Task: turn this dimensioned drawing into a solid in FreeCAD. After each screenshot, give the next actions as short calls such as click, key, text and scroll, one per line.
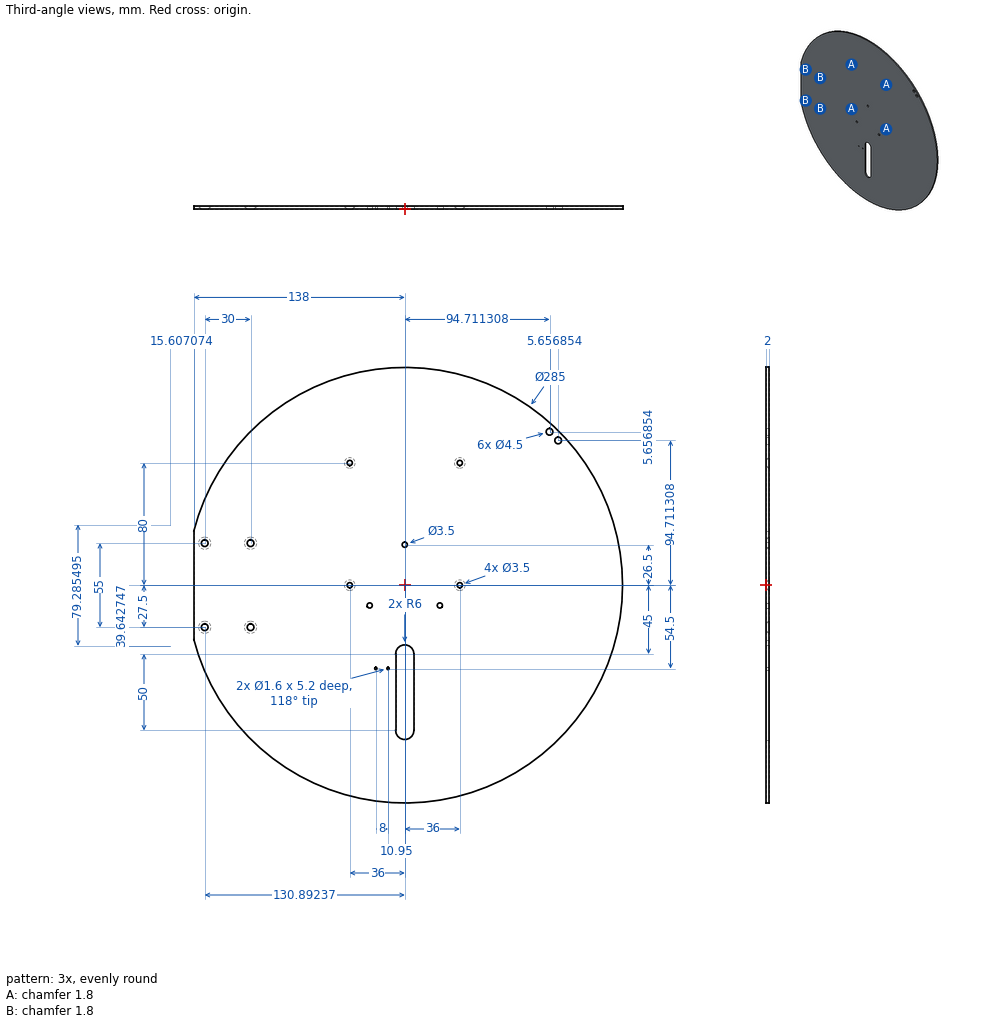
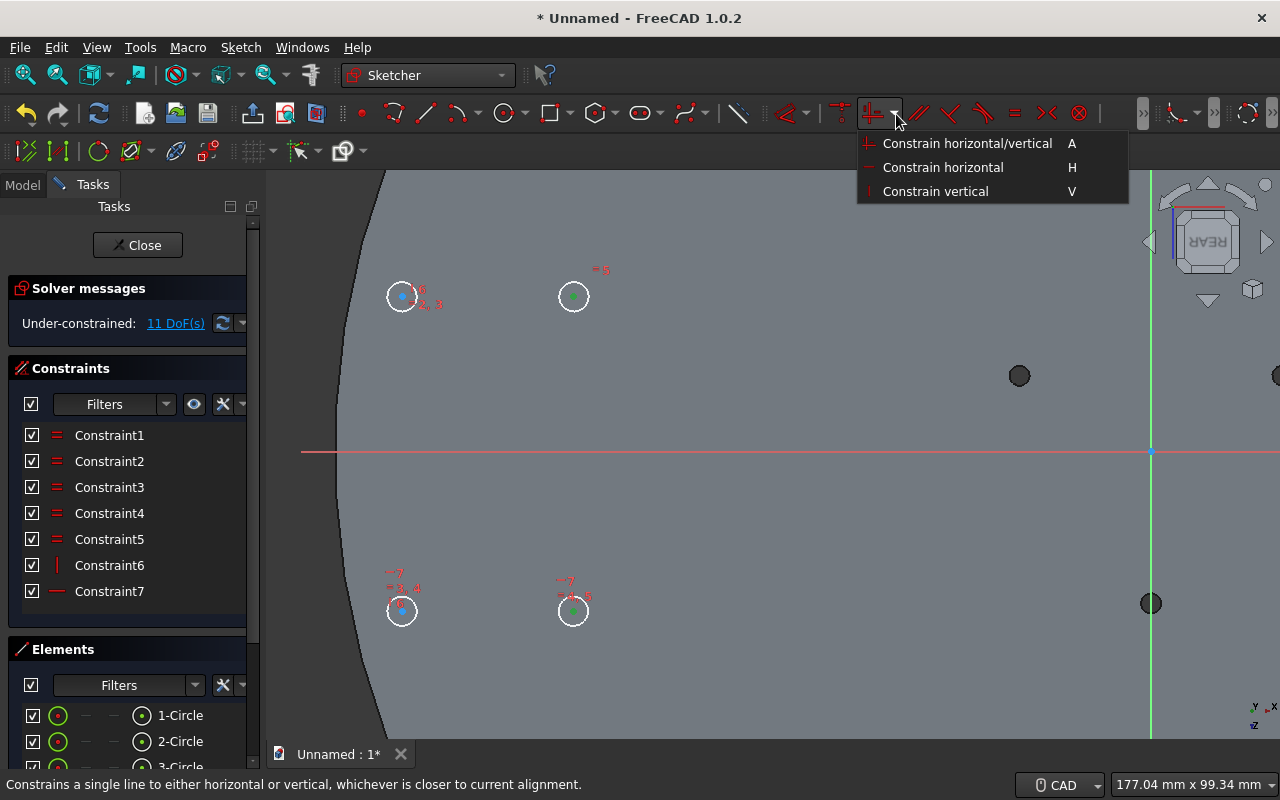
click(993, 191)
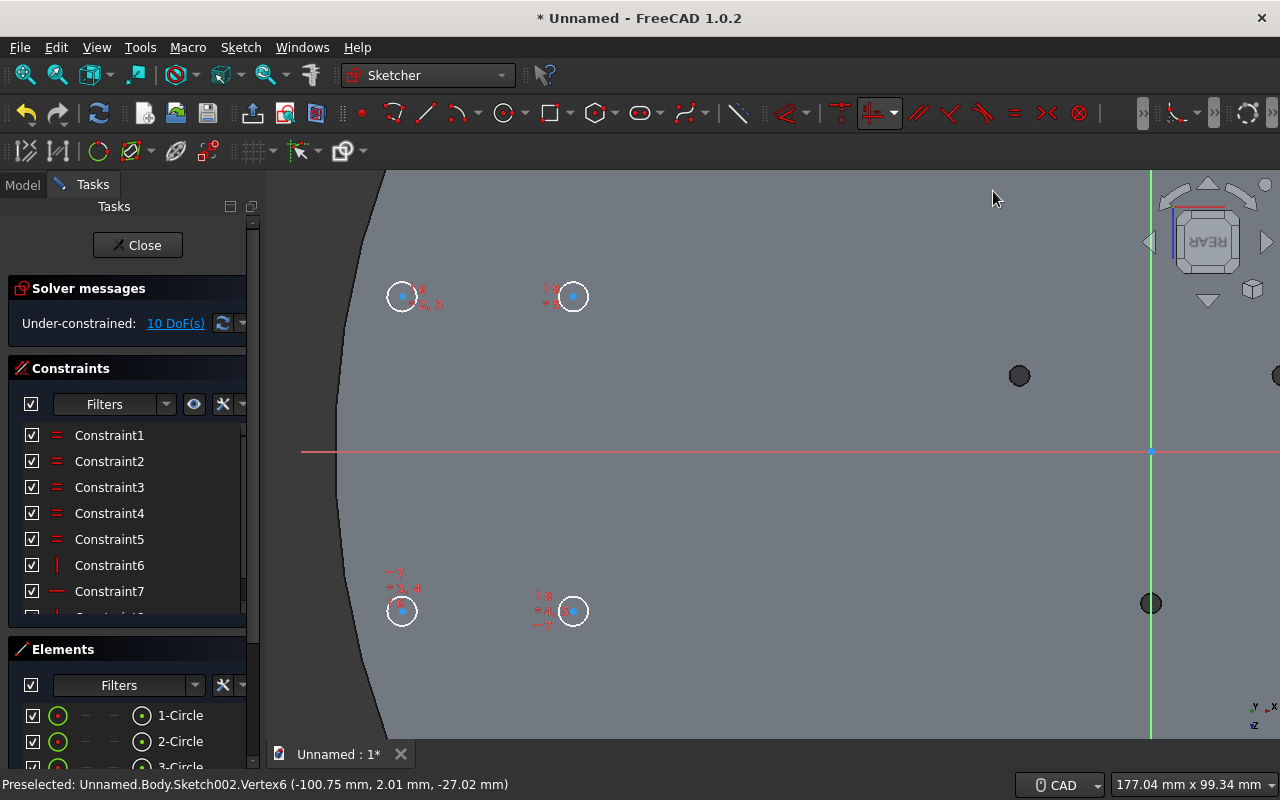
click(402, 297)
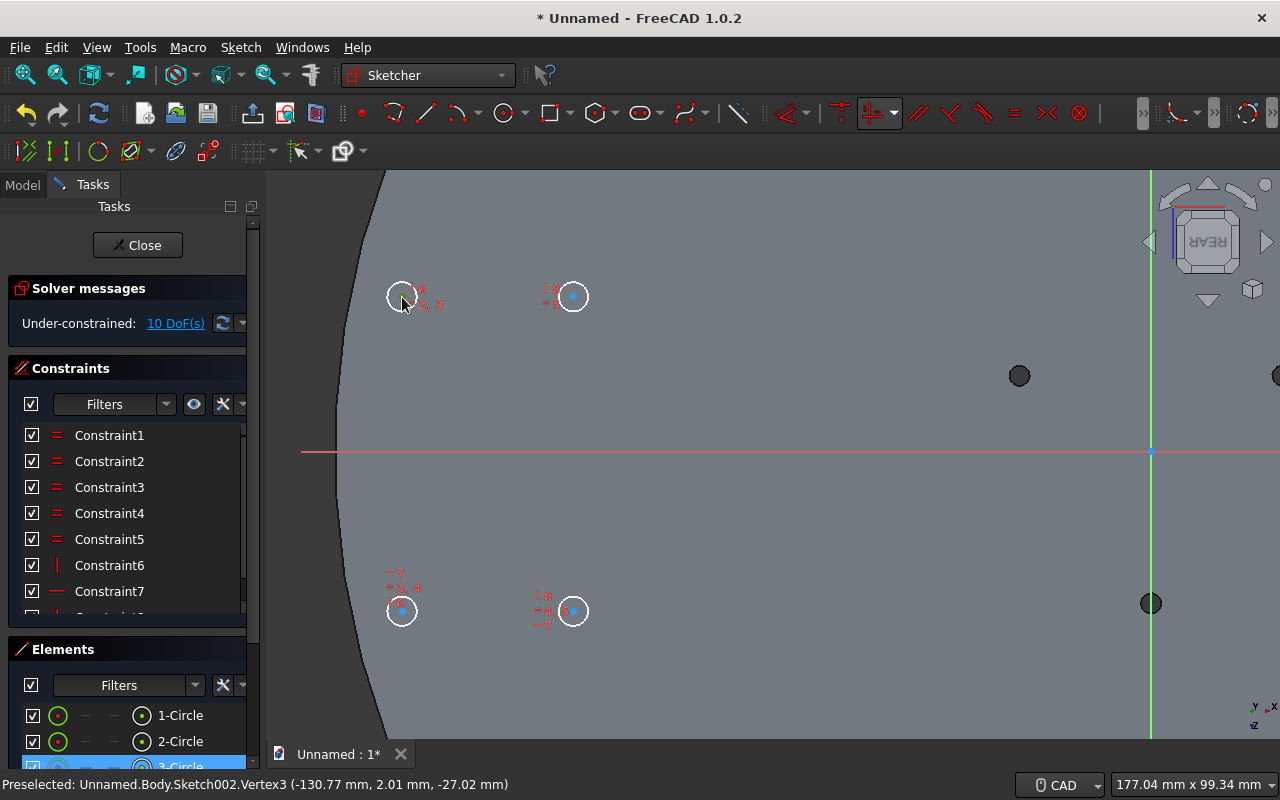
click(573, 297)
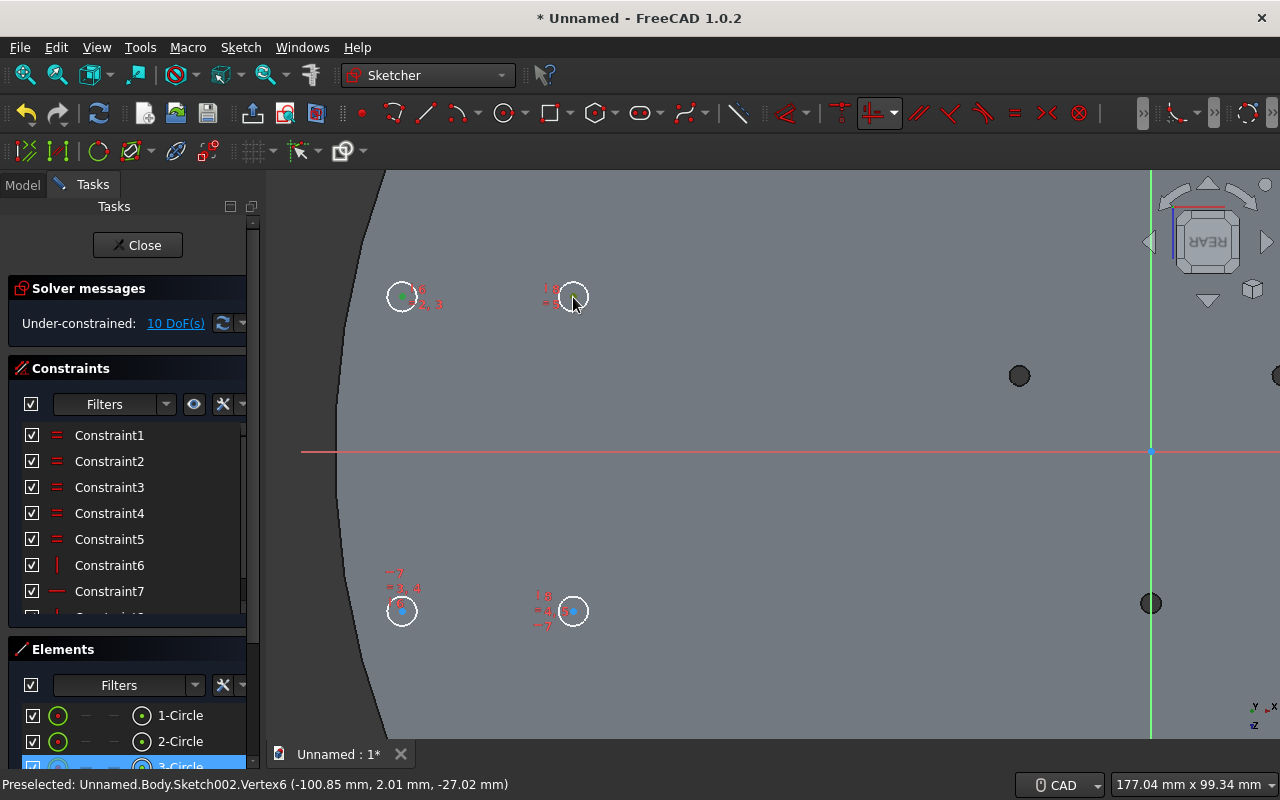
click(896, 114)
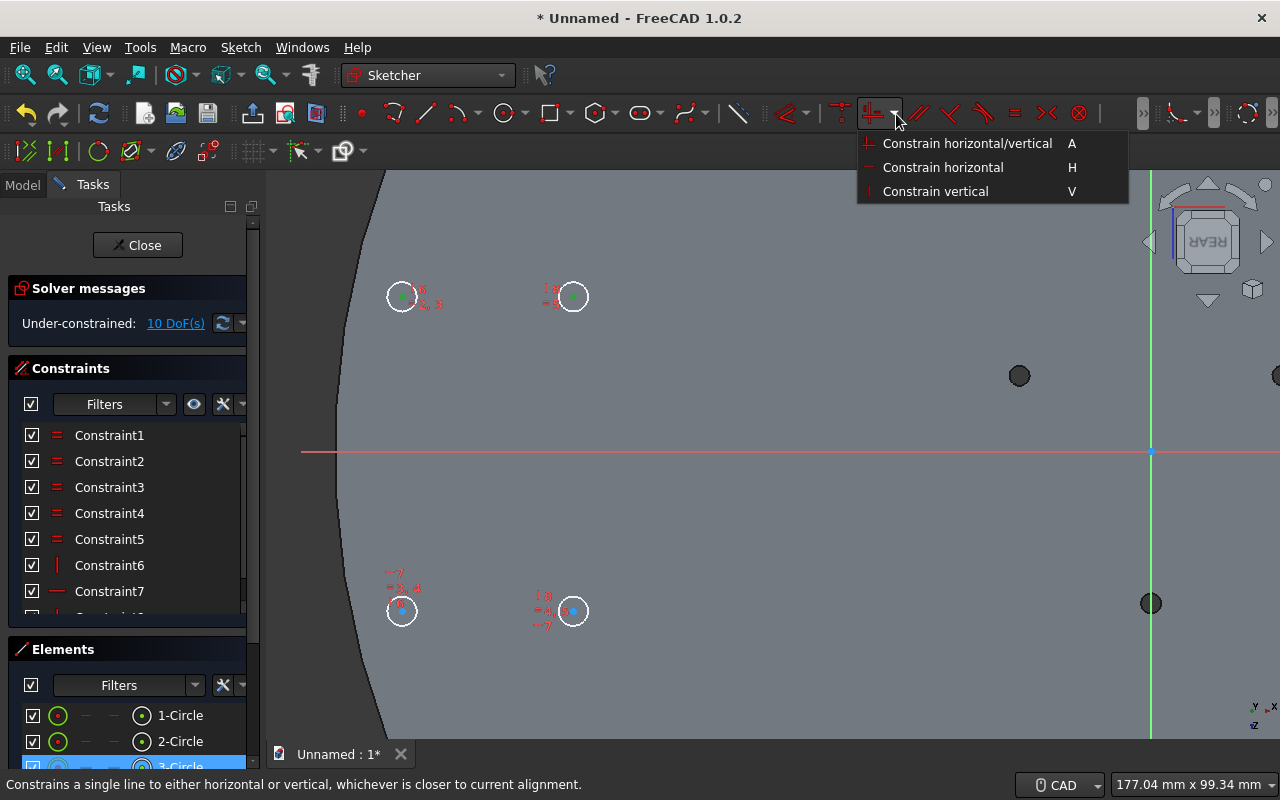
click(993, 167)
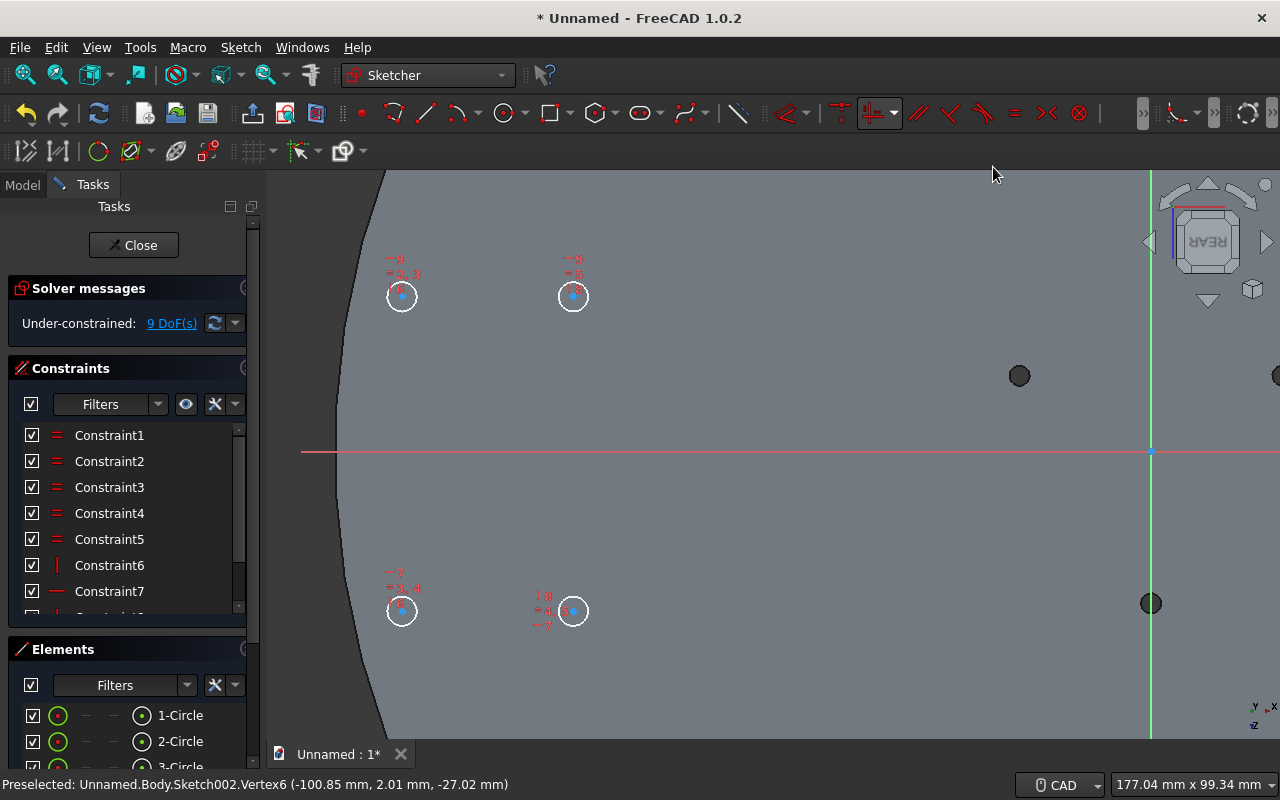
click(786, 114)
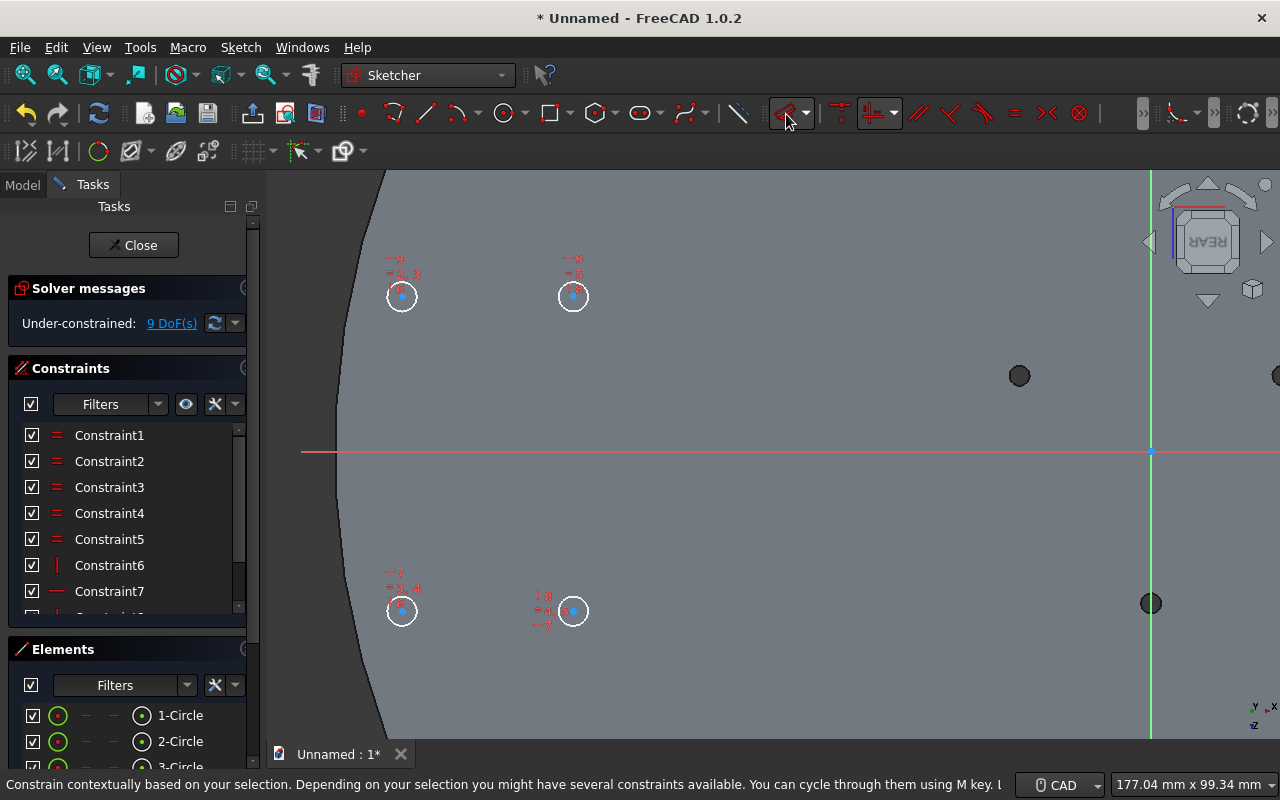
scroll(411, 287, down, 4)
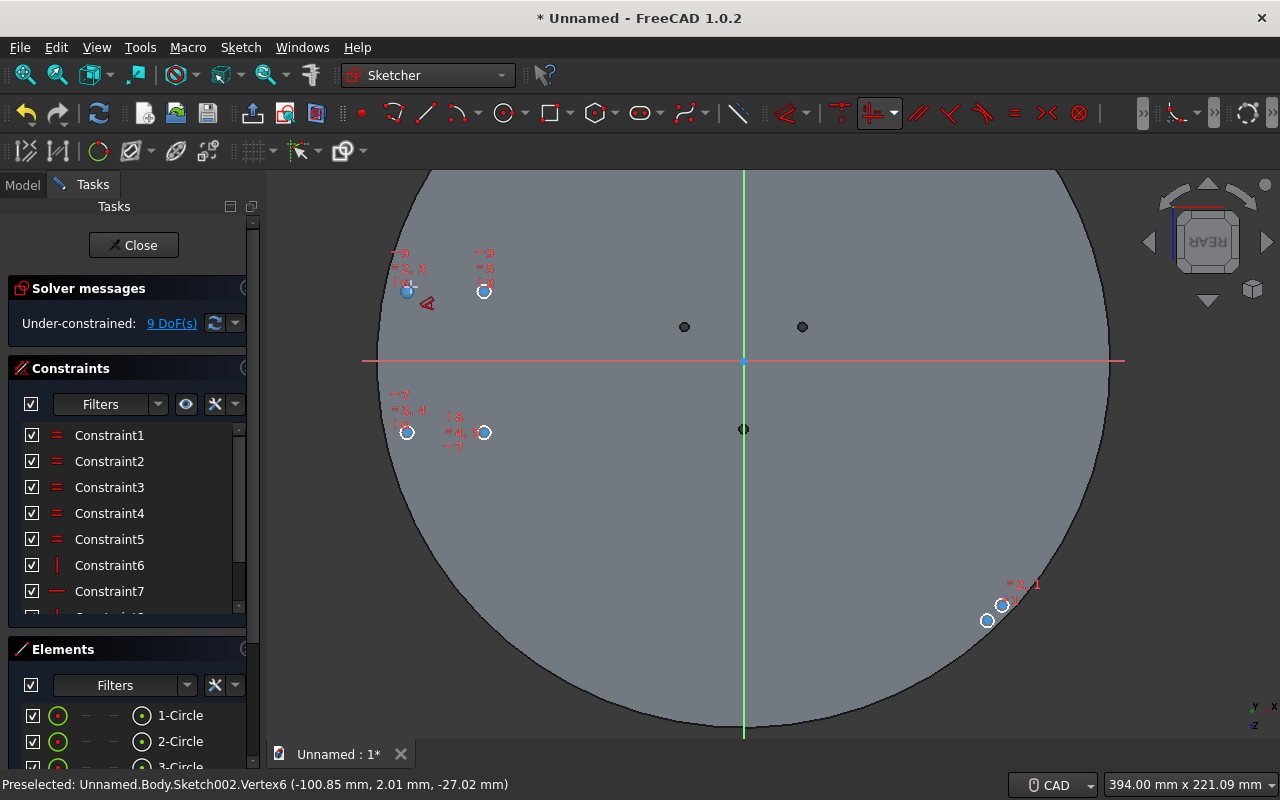
scroll(992, 616, up, 7)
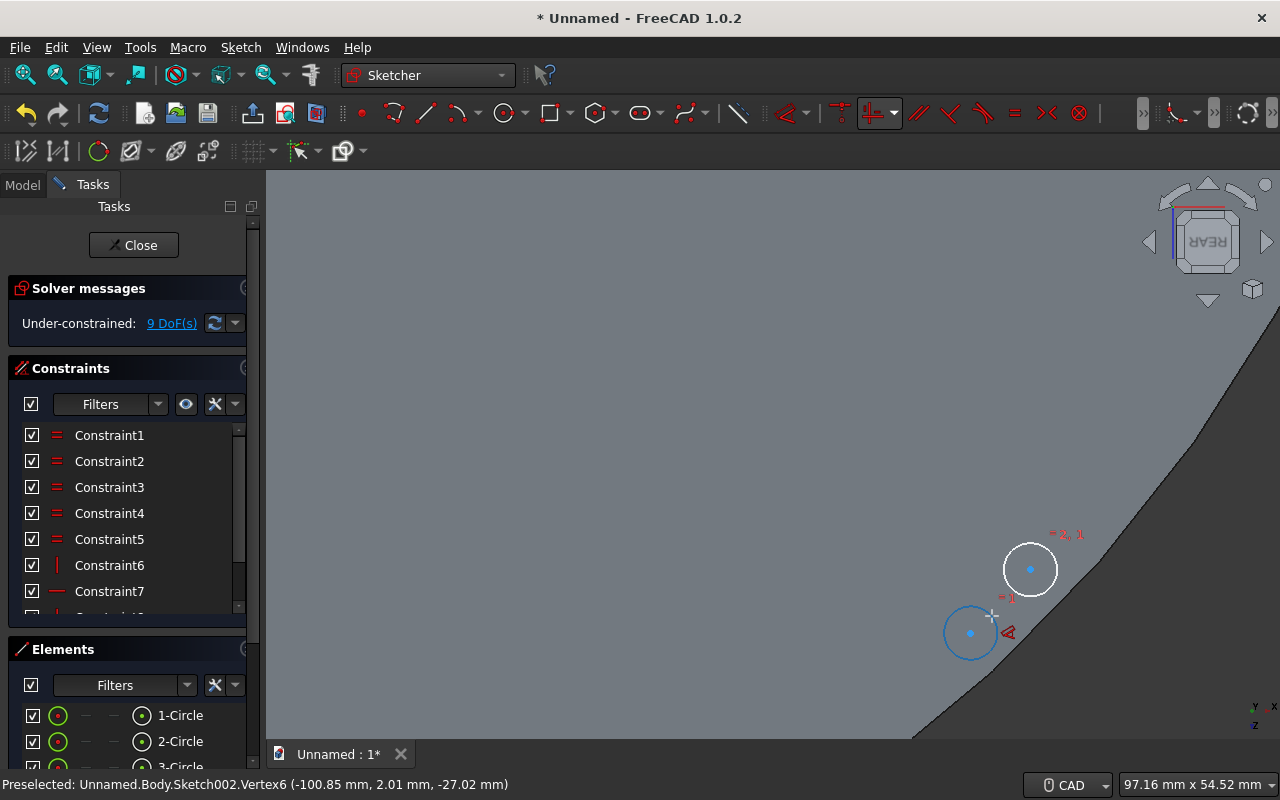
click(990, 614)
click(1028, 617)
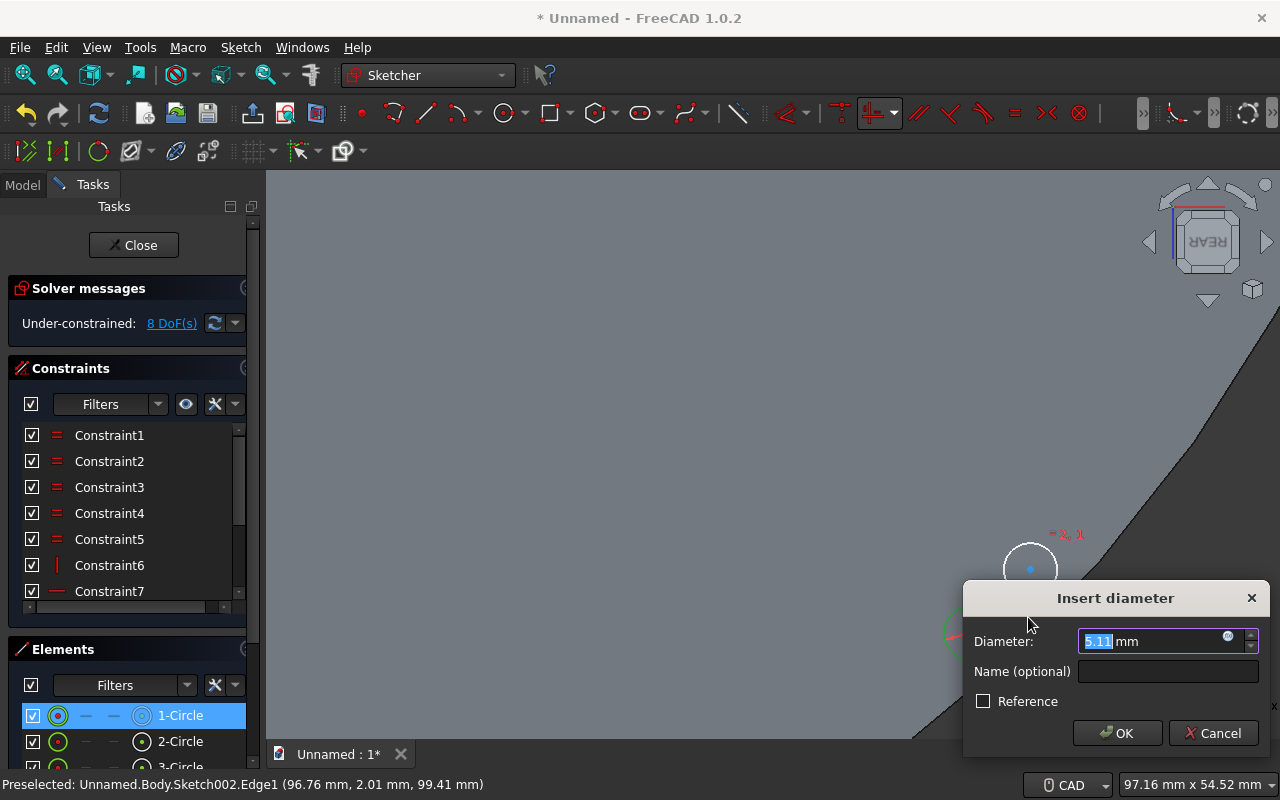
text(4.5)
key(Return)